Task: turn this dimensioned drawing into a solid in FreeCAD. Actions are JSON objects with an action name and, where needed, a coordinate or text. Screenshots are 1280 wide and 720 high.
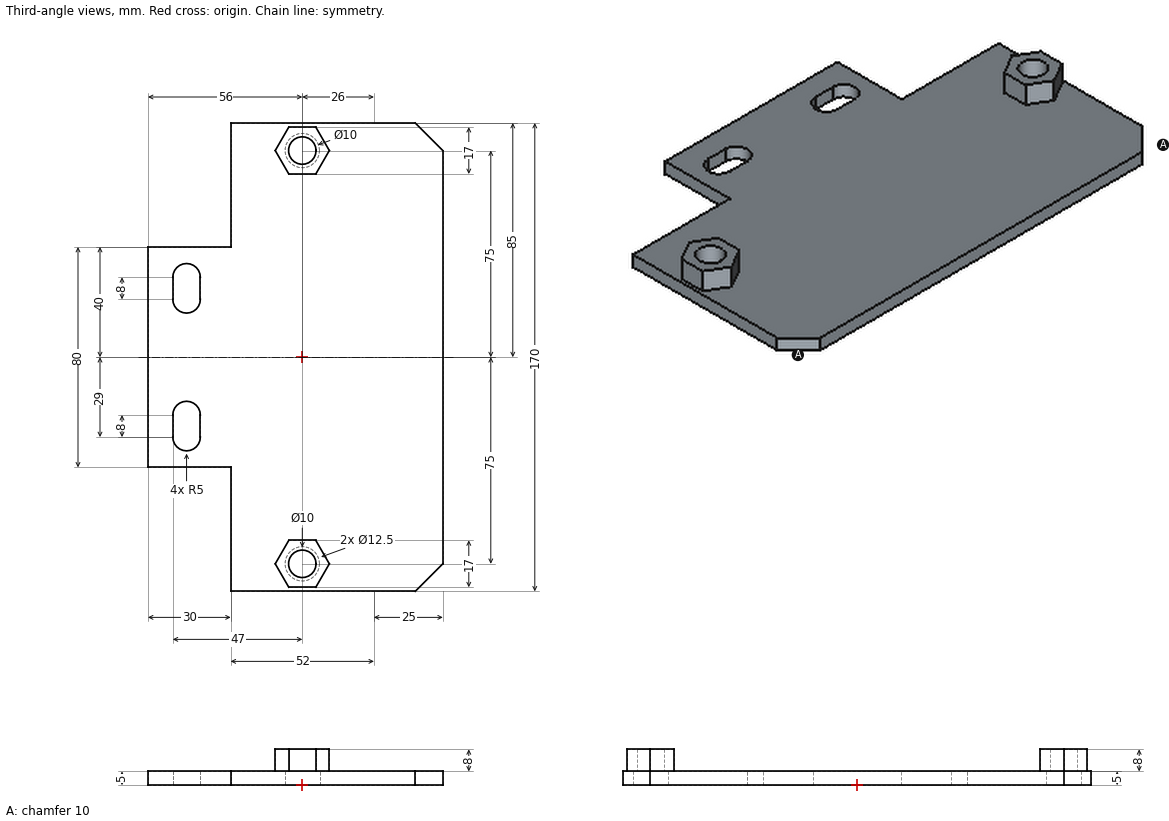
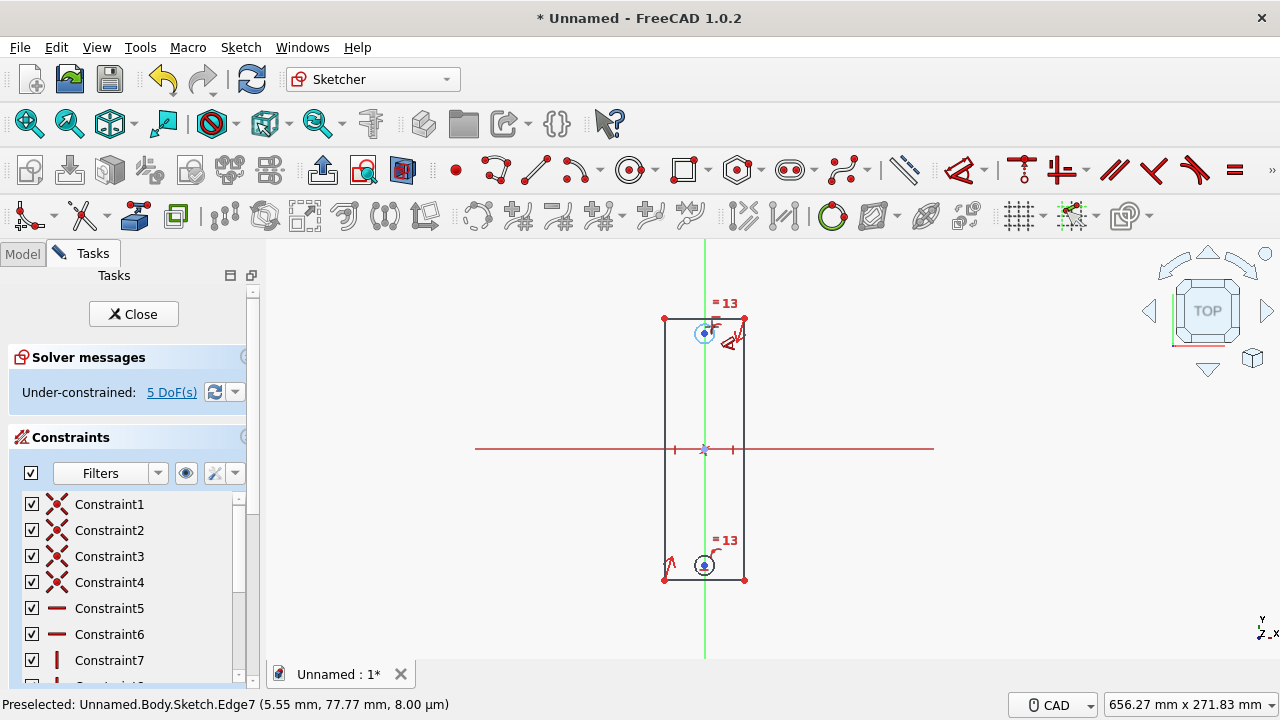
{"action": "scroll", "coordinate": [711, 559], "scroll_direction": "up", "scroll_amount": 4}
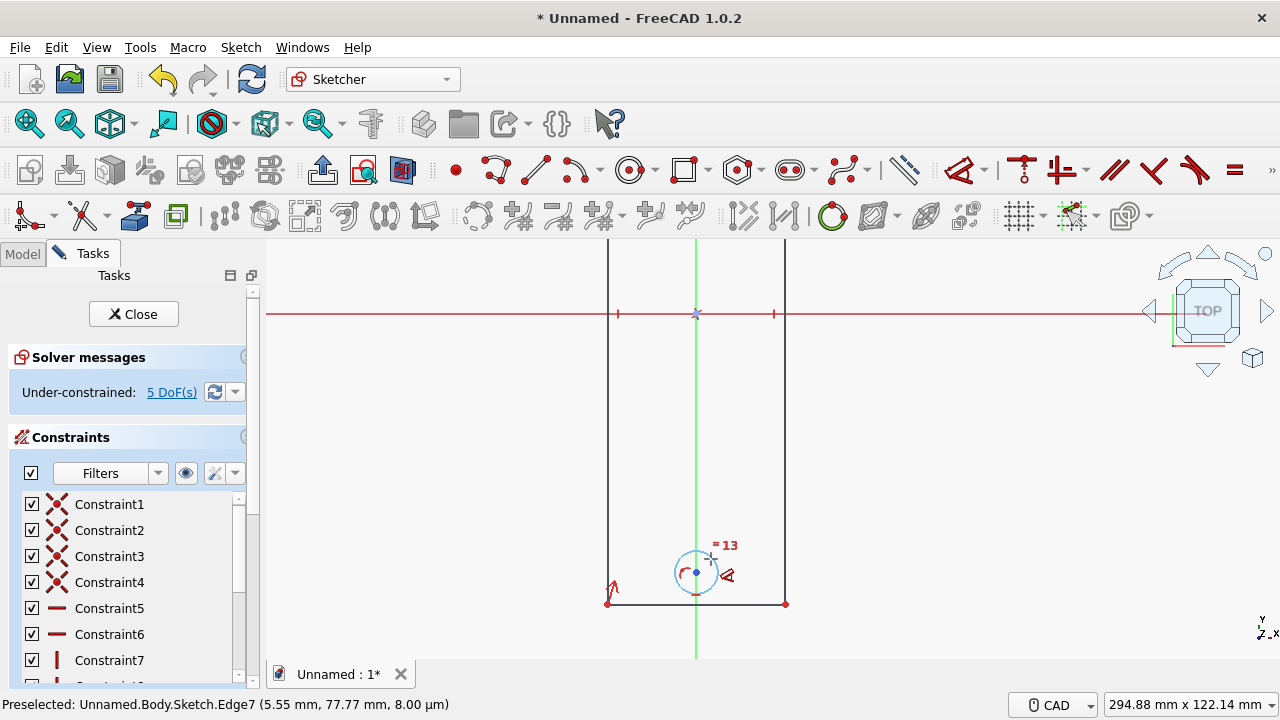
{"action": "left_click", "coordinate": [711, 557]}
{"action": "left_click", "coordinate": [733, 534]}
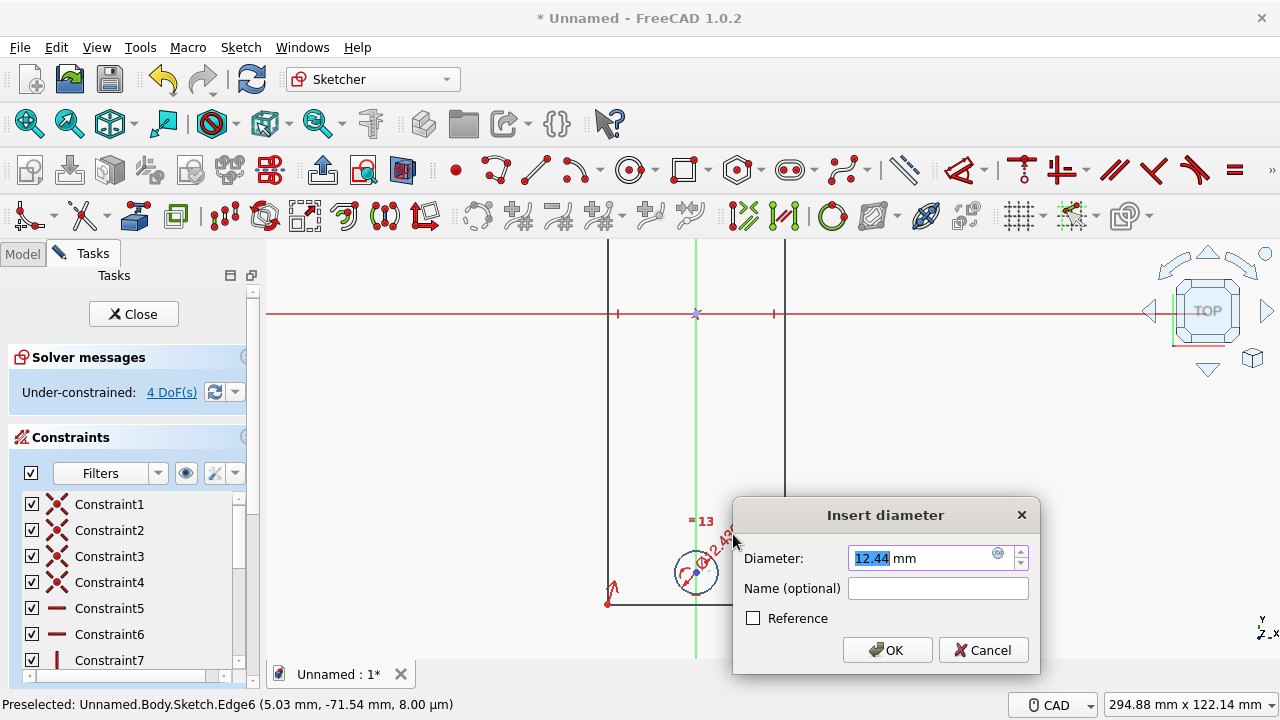
{"action": "type", "text": "12.5"}
{"action": "key", "text": "Return"}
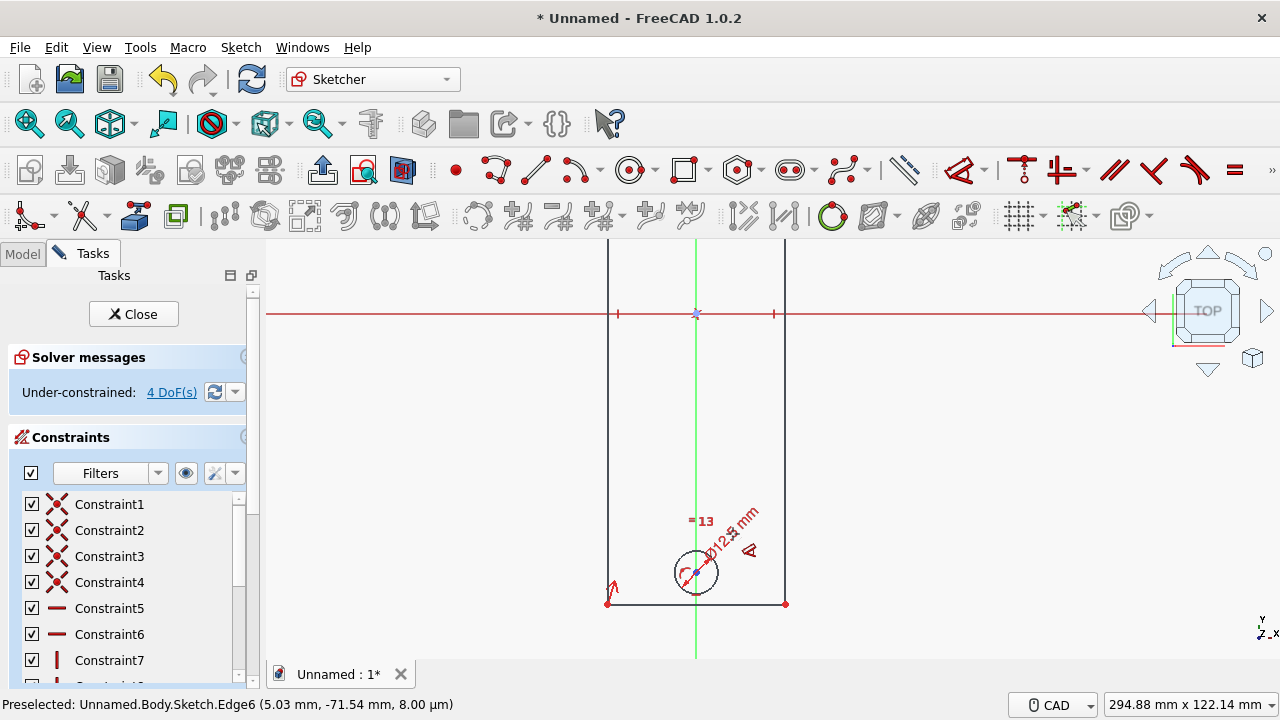
{"action": "left_click", "coordinate": [661, 605]}
{"action": "left_click", "coordinate": [656, 571]}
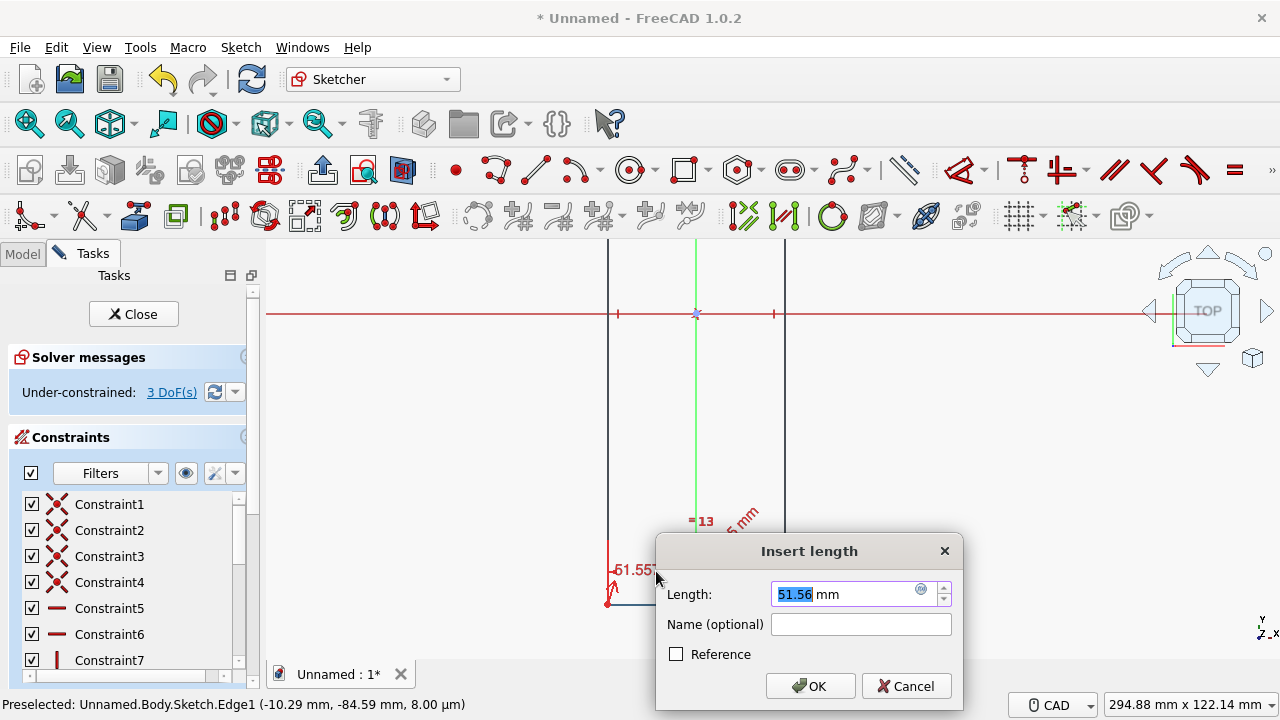
{"action": "type", "text": "52"}
{"action": "key", "text": "Return"}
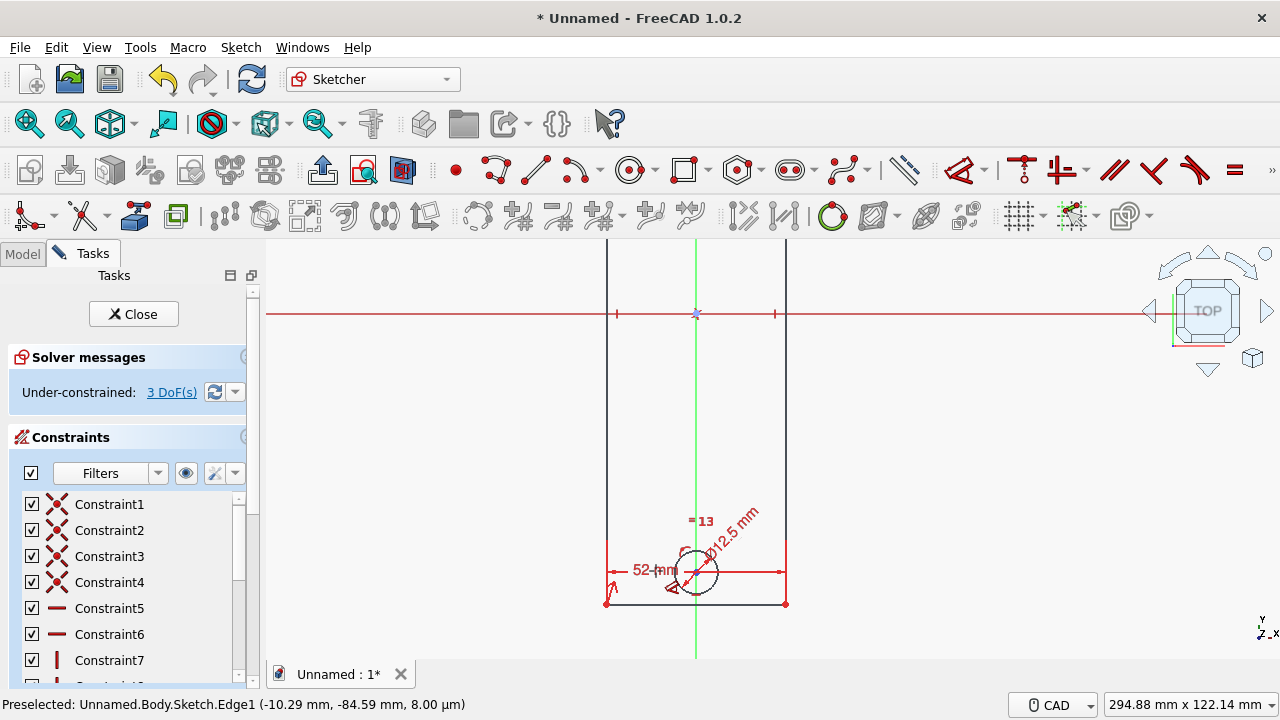
{"action": "left_click", "coordinate": [696, 573]}
{"action": "left_click", "coordinate": [730, 443]}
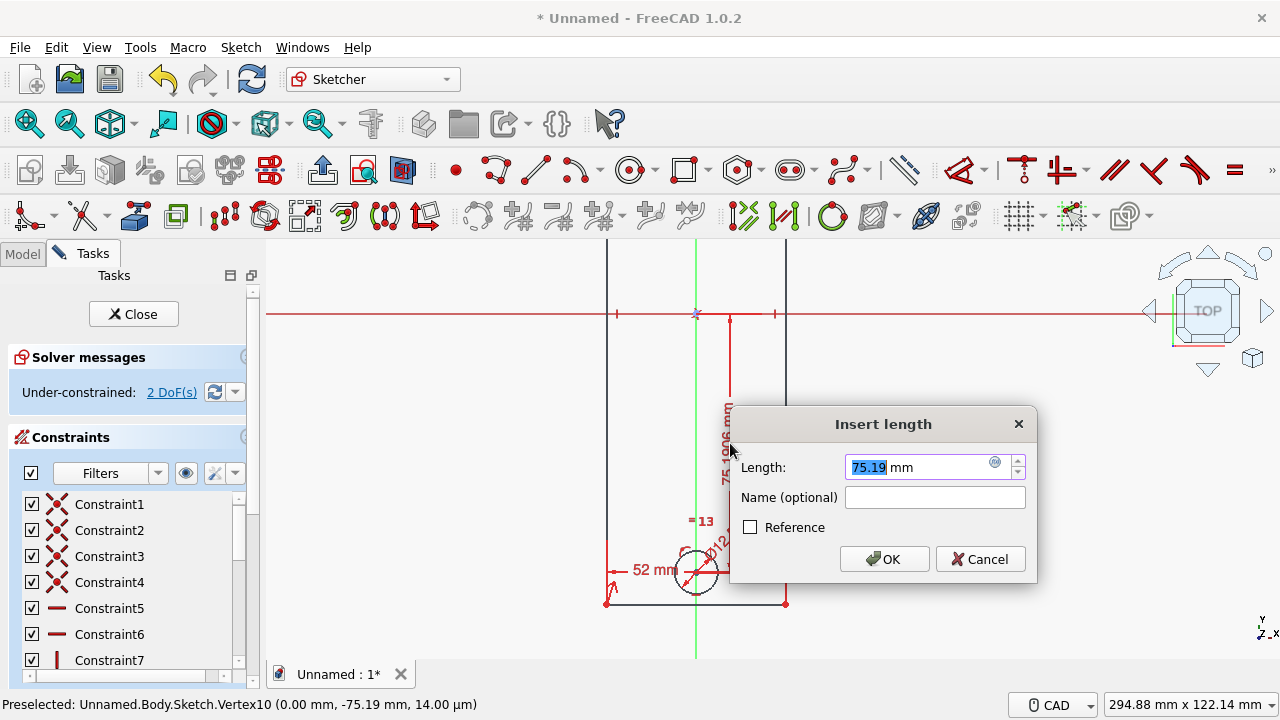
{"action": "type", "text": "75"}
{"action": "key", "text": "Return"}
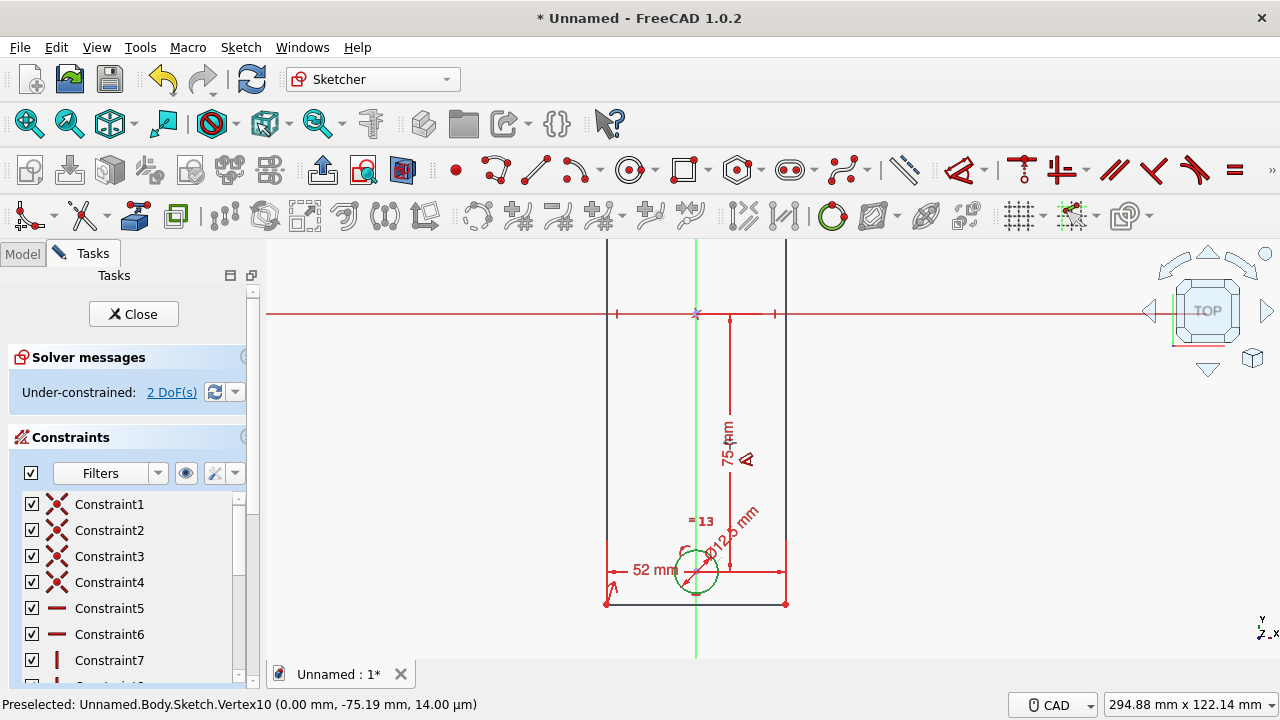
{"action": "scroll", "coordinate": [711, 559], "scroll_direction": "down", "scroll_amount": 4}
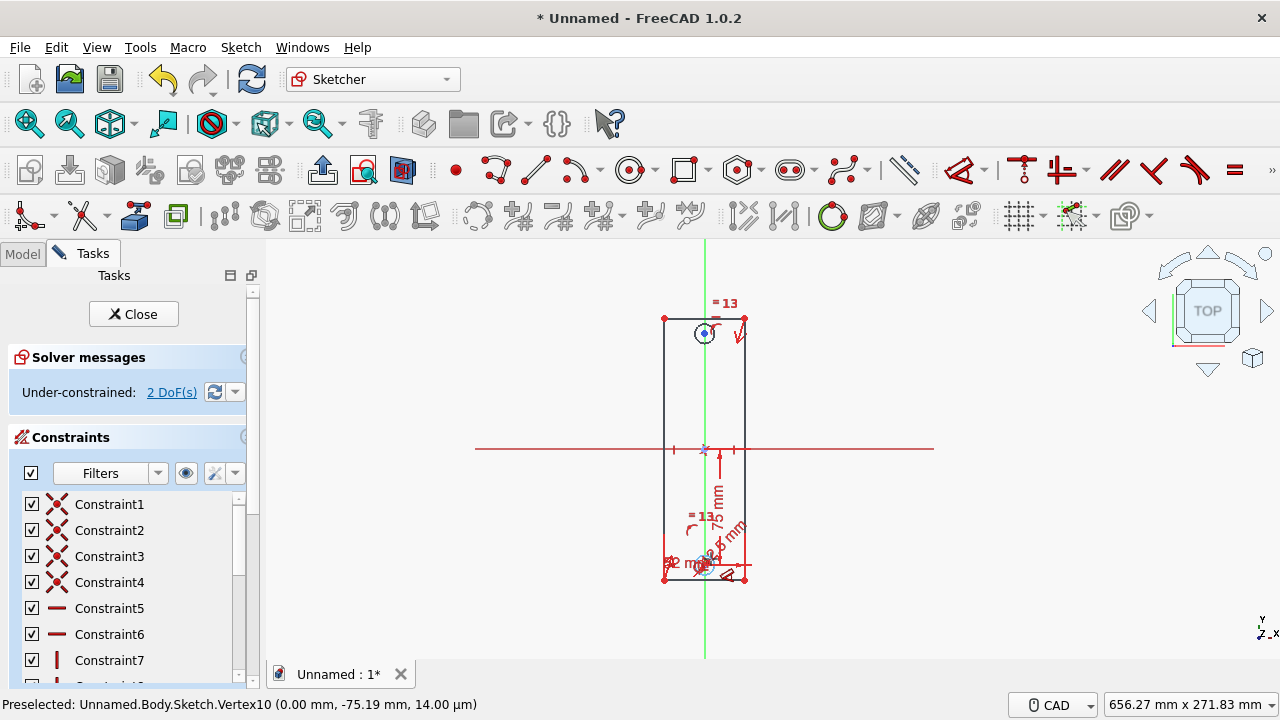
{"action": "left_click", "coordinate": [705, 334]}
{"action": "left_click", "coordinate": [763, 392]}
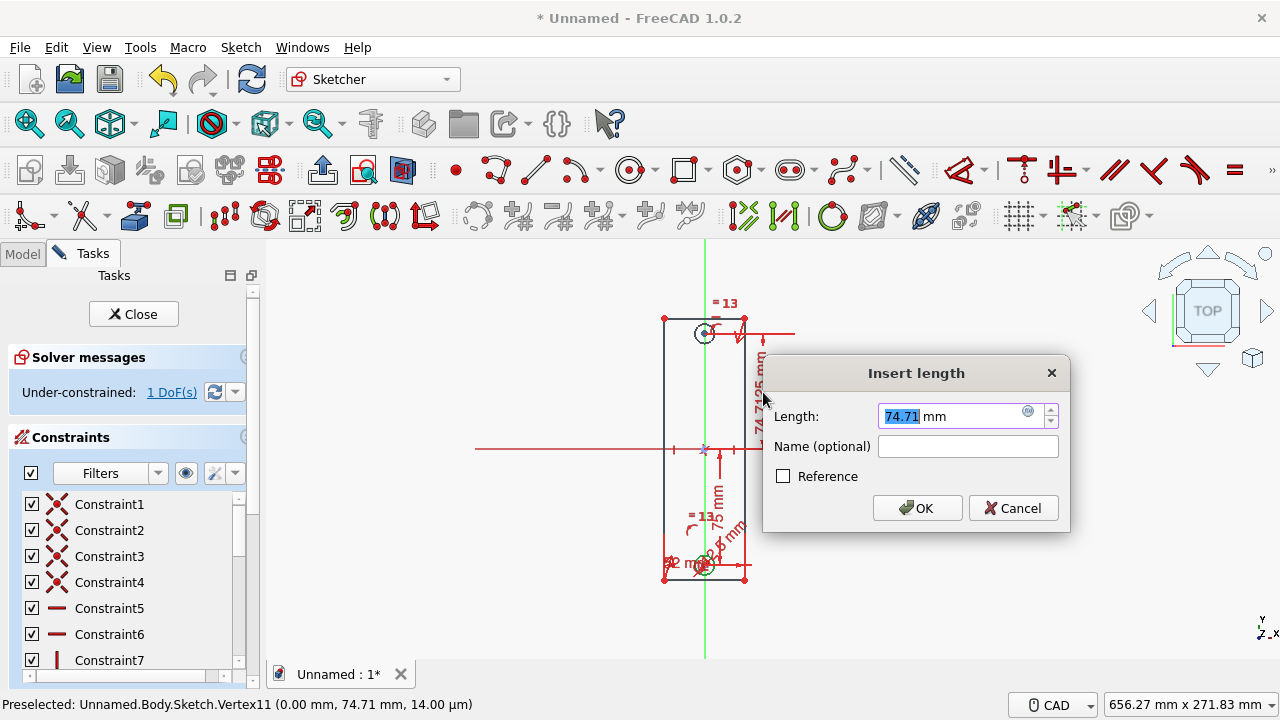
{"action": "type", "text": "75"}
{"action": "key", "text": "Return"}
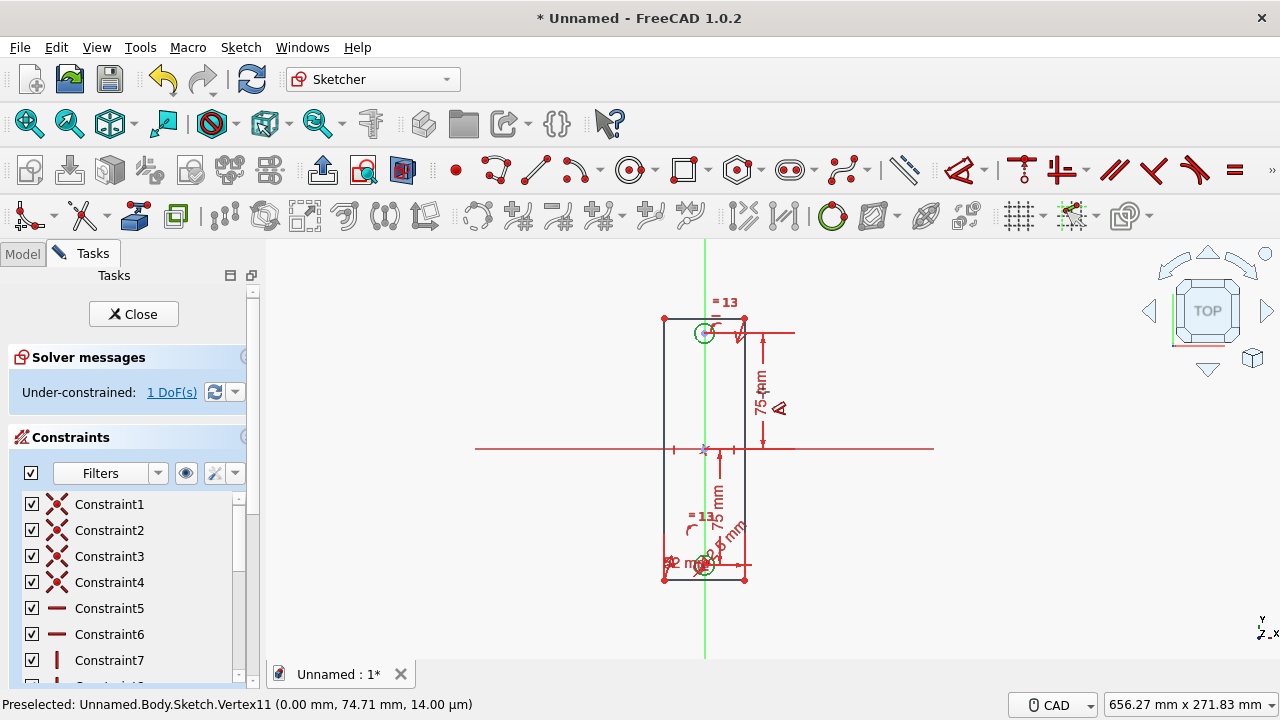
{"action": "left_click", "coordinate": [745, 502]}
{"action": "left_click", "coordinate": [779, 358]}